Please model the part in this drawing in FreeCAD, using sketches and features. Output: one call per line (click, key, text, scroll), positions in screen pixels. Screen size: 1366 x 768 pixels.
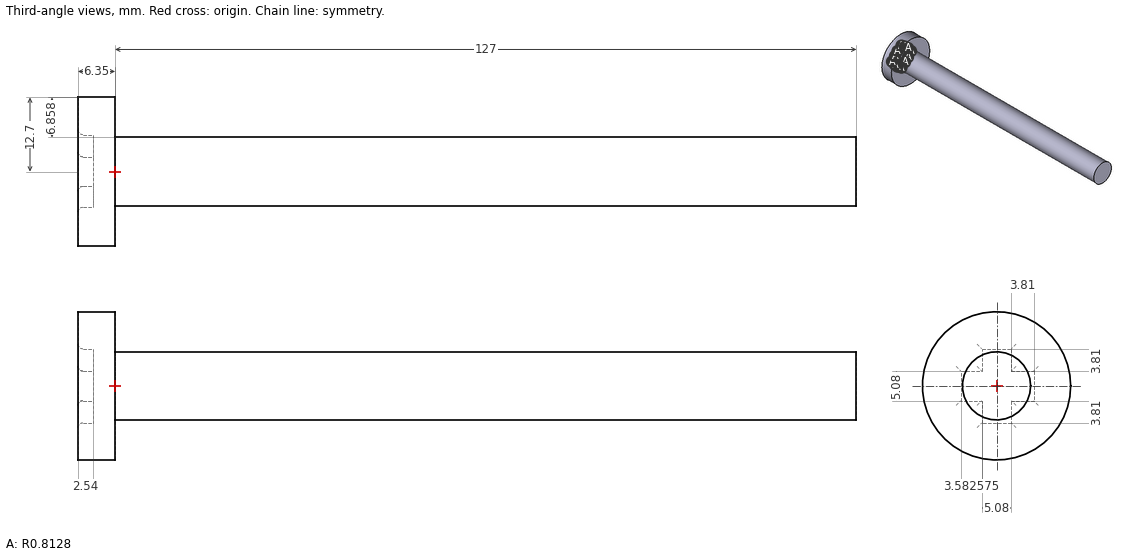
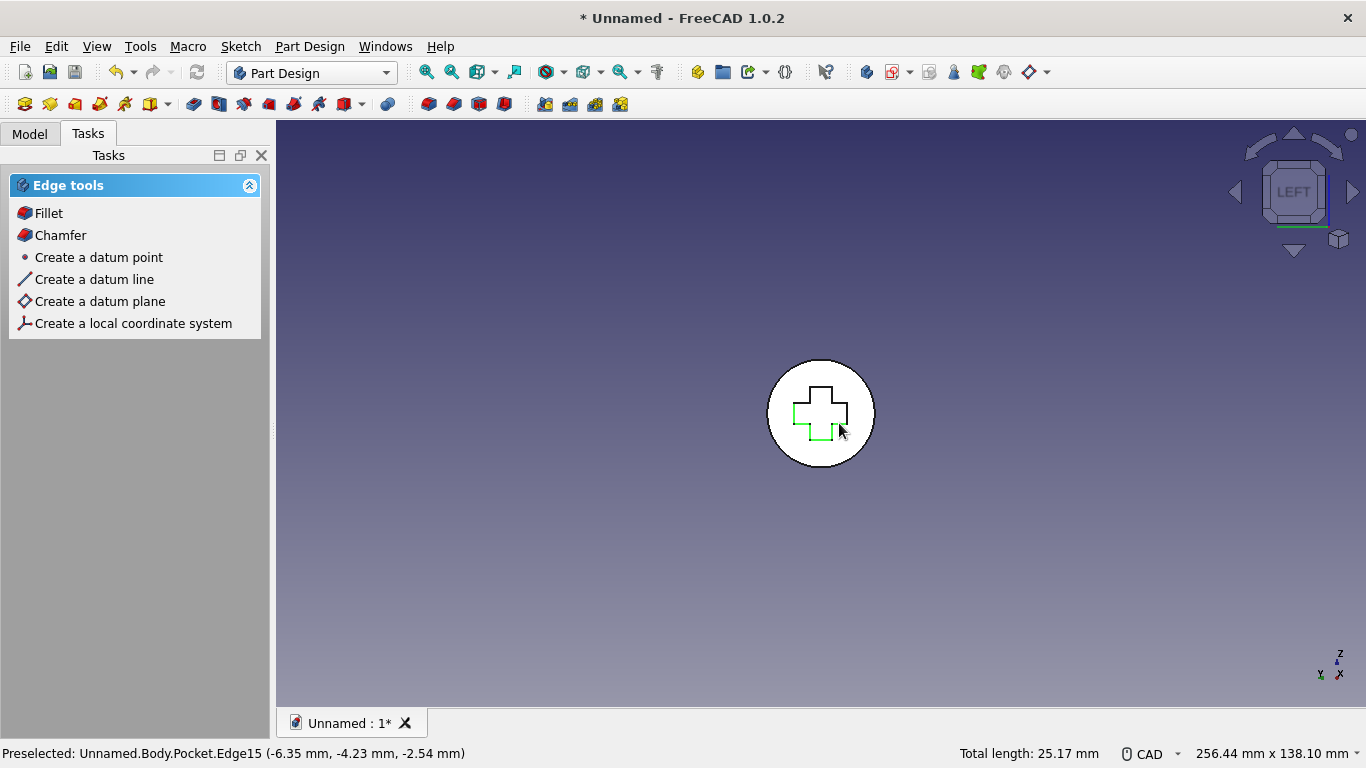
click(847, 412, ctrl)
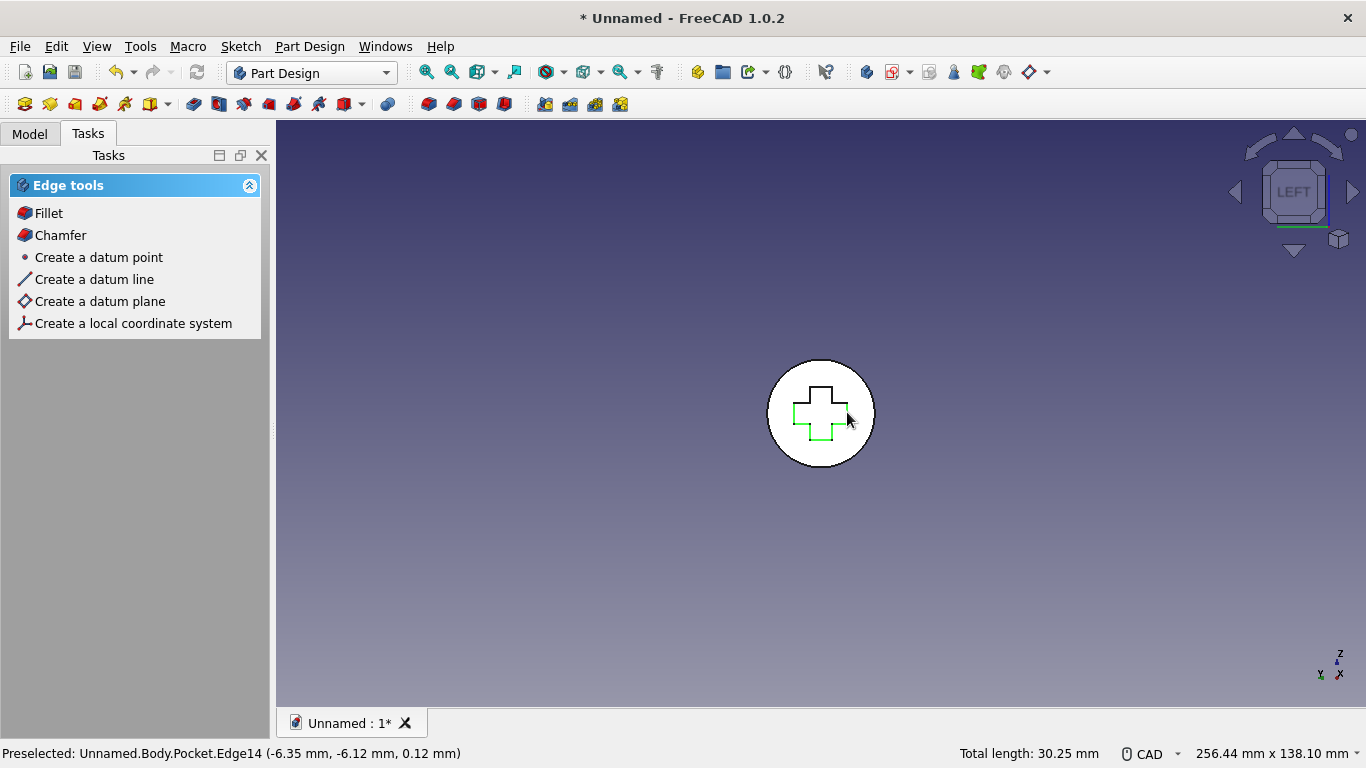
click(839, 402, ctrl)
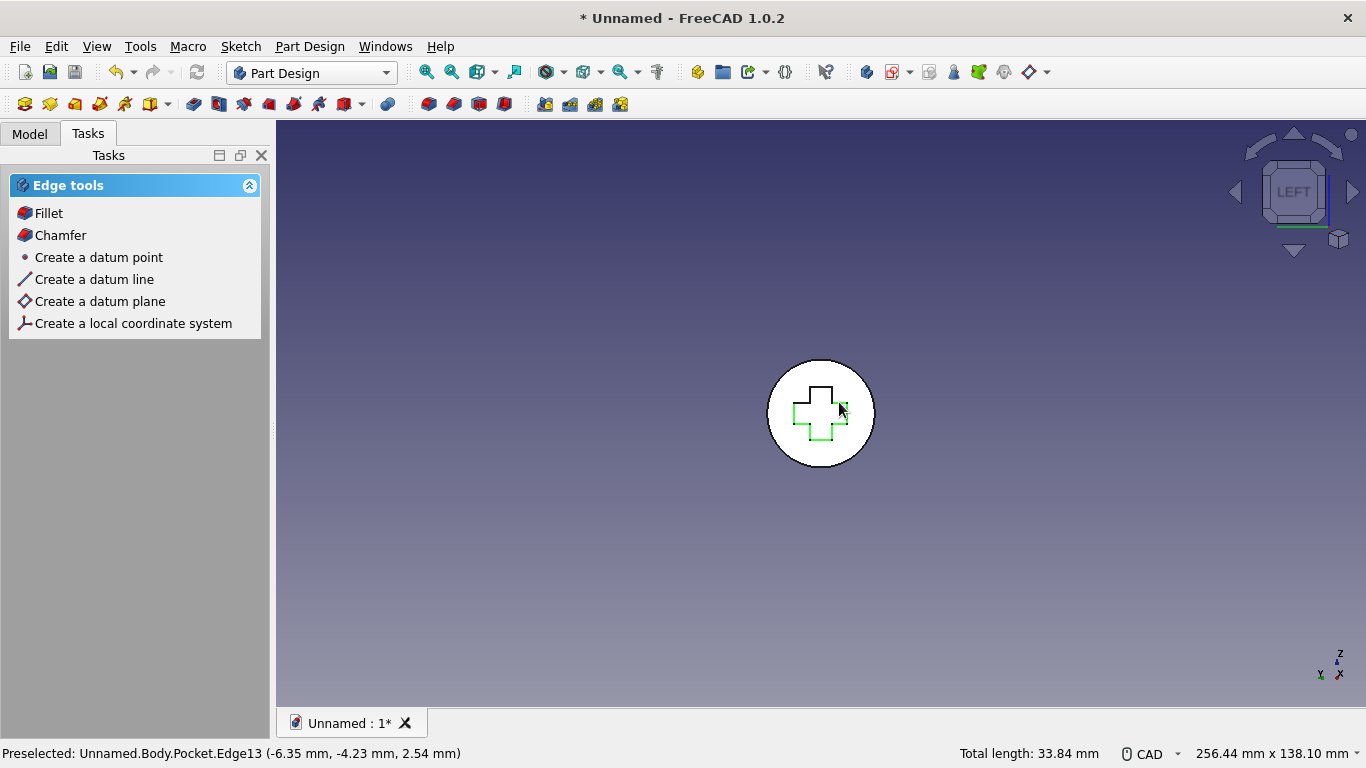
click(832, 394, ctrl)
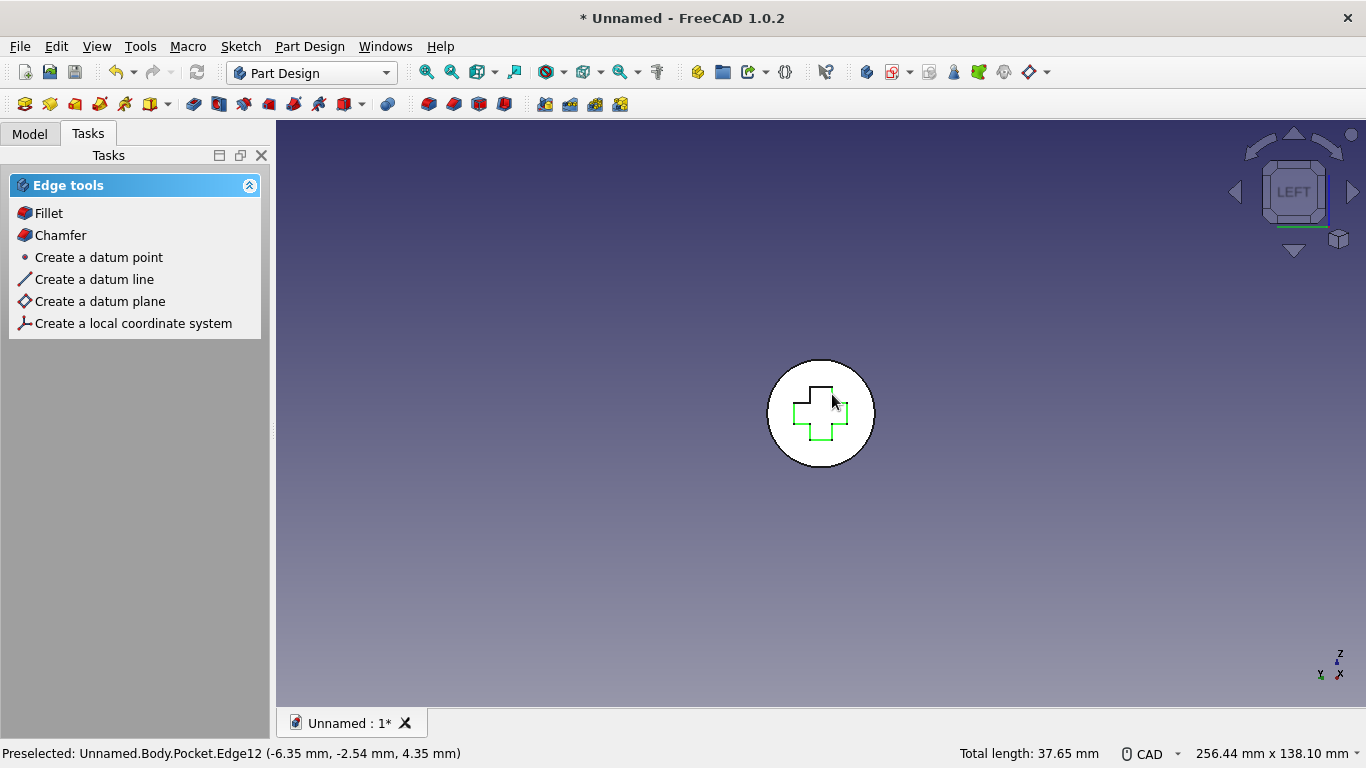
click(821, 386, ctrl)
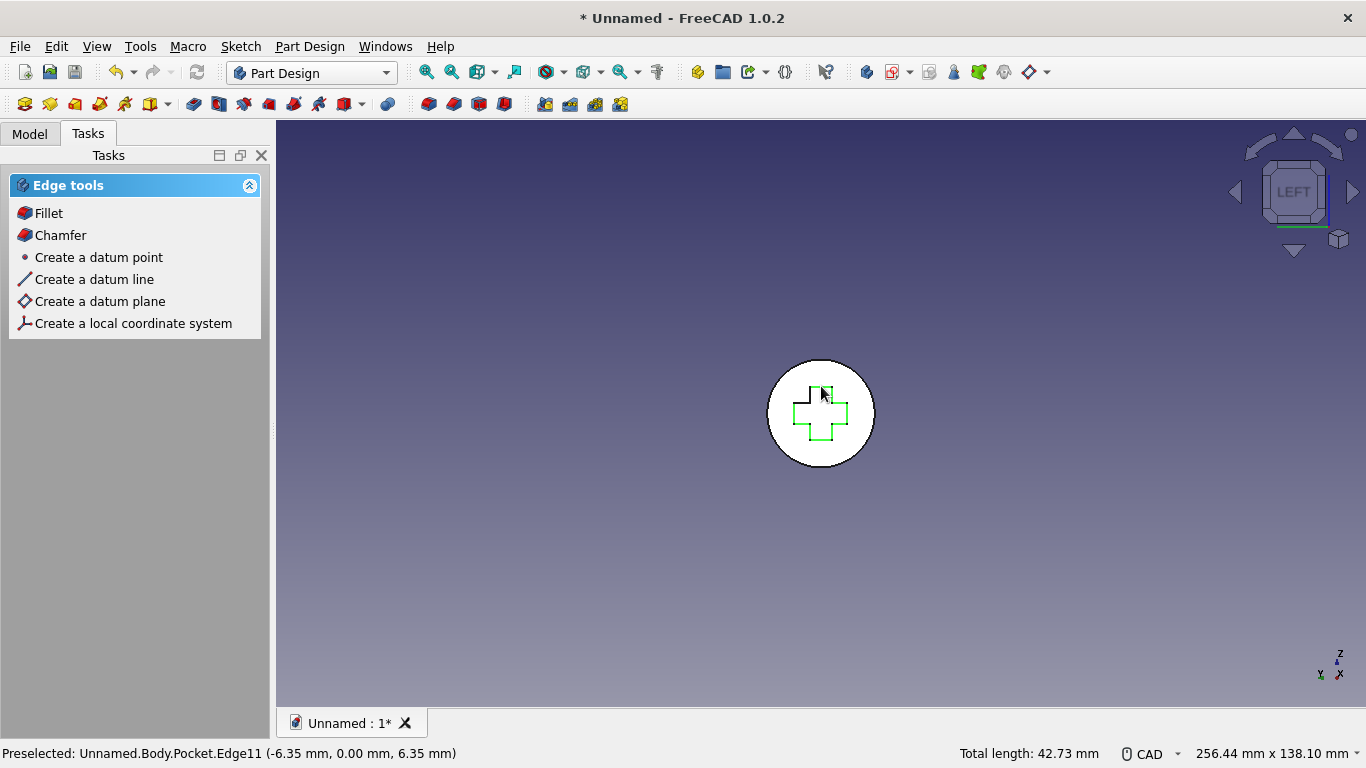
click(810, 394, ctrl)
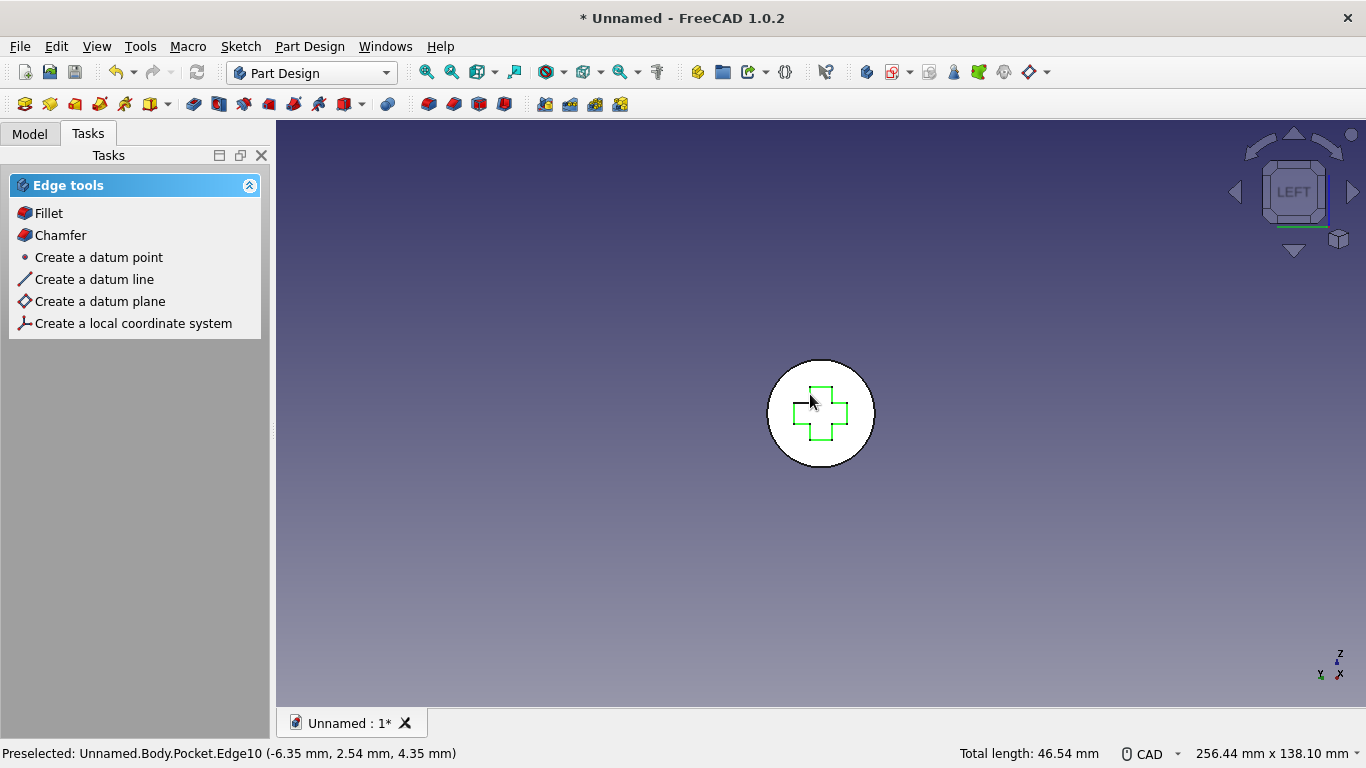
click(802, 402, ctrl)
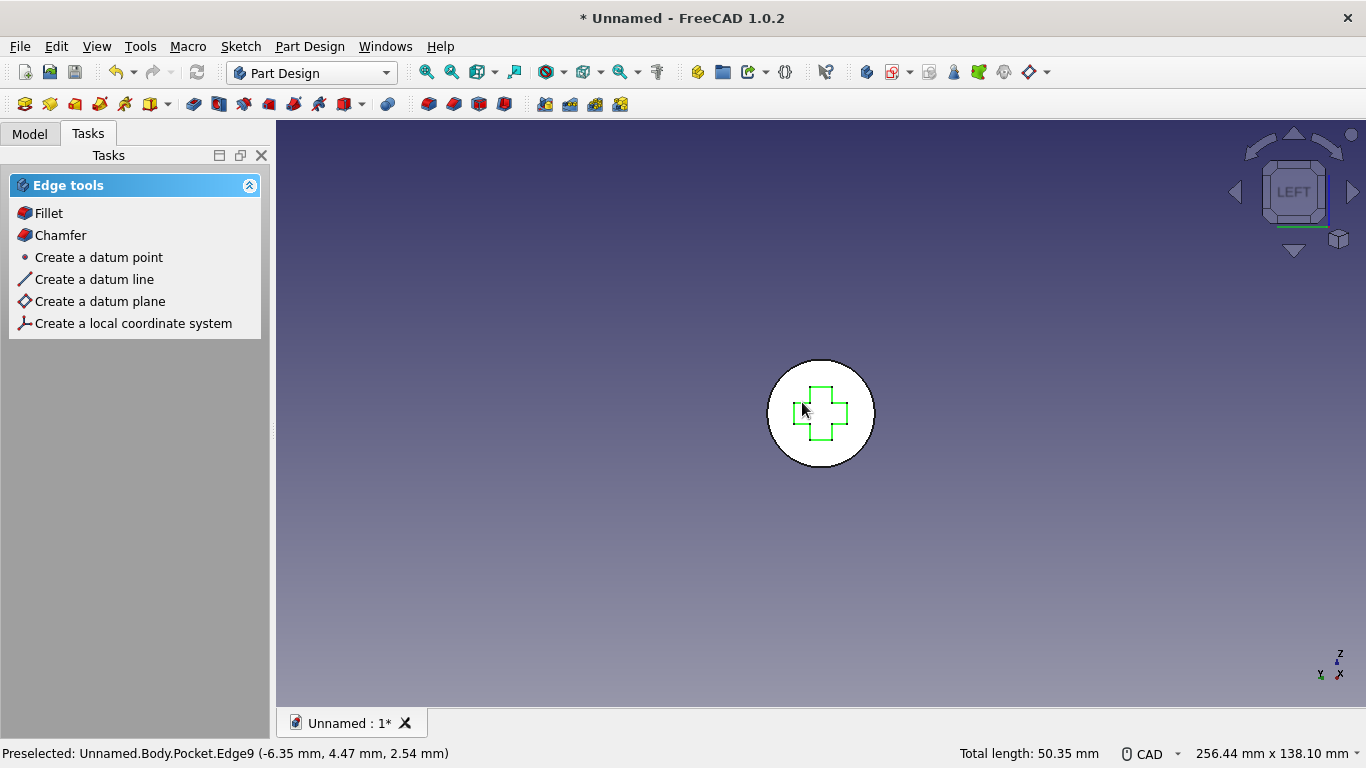
click(429, 104)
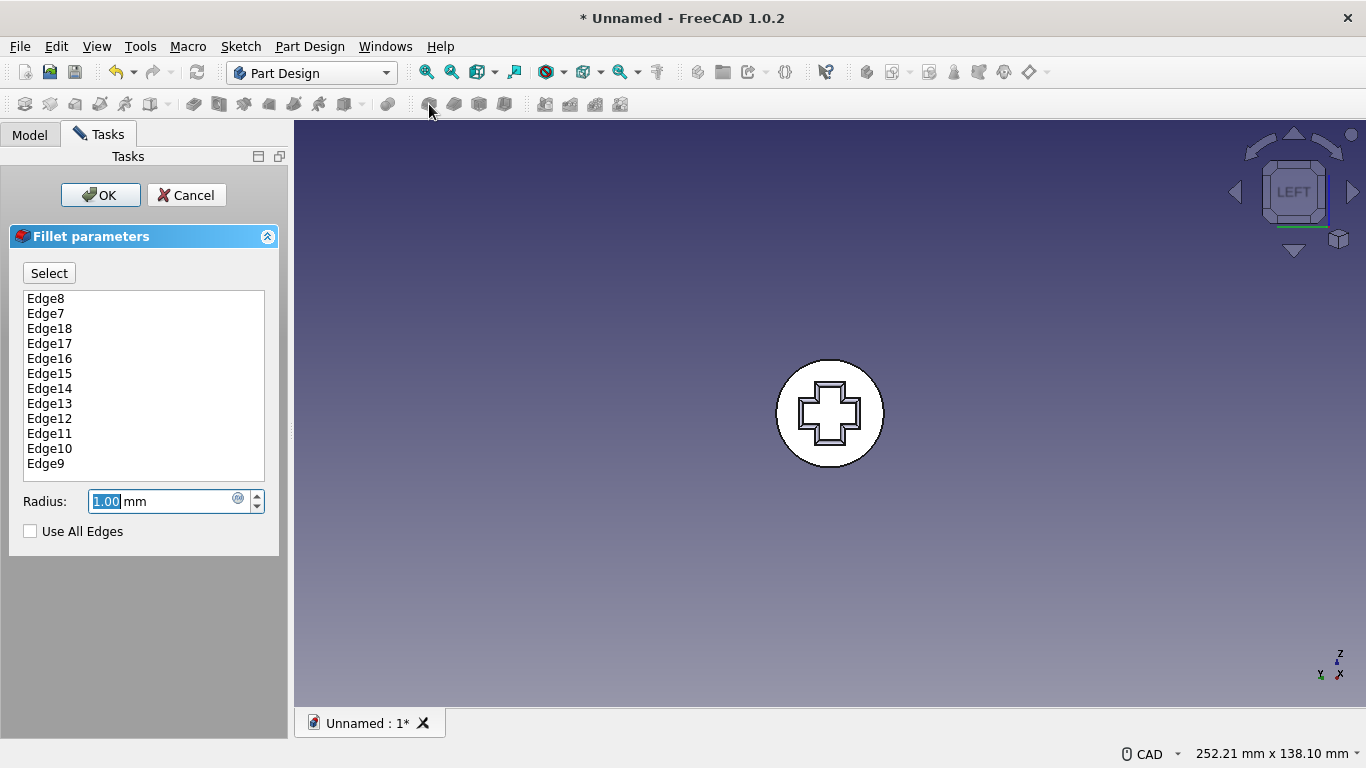
text(0.8128)
key(Tab)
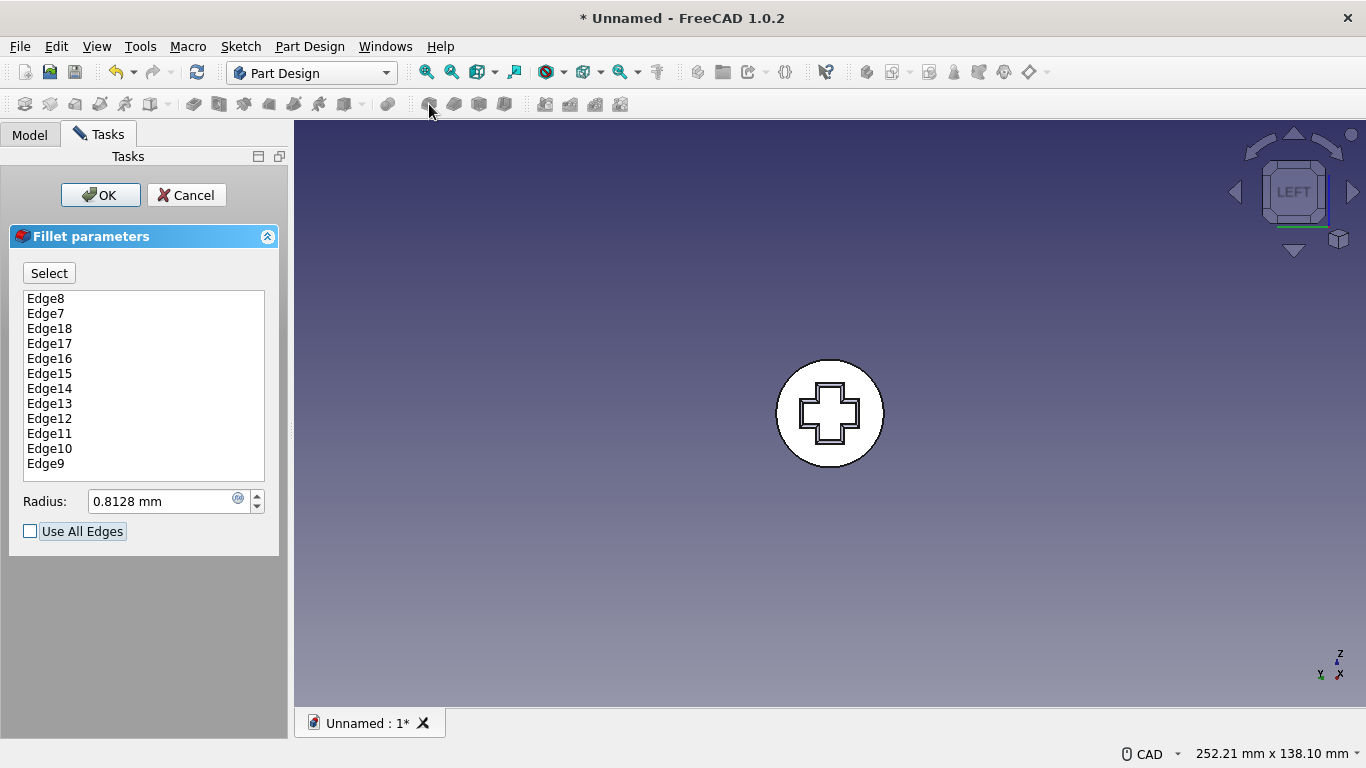
click(101, 195)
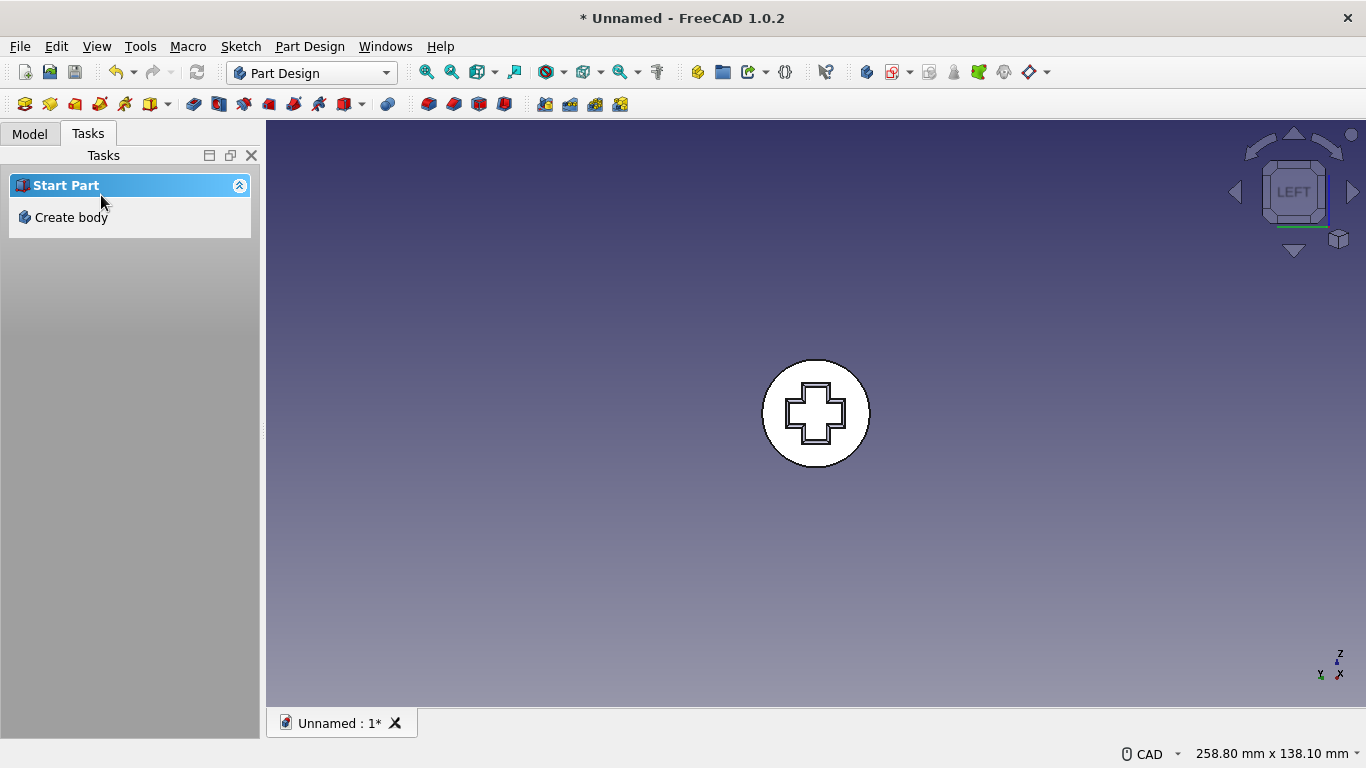
key(0)